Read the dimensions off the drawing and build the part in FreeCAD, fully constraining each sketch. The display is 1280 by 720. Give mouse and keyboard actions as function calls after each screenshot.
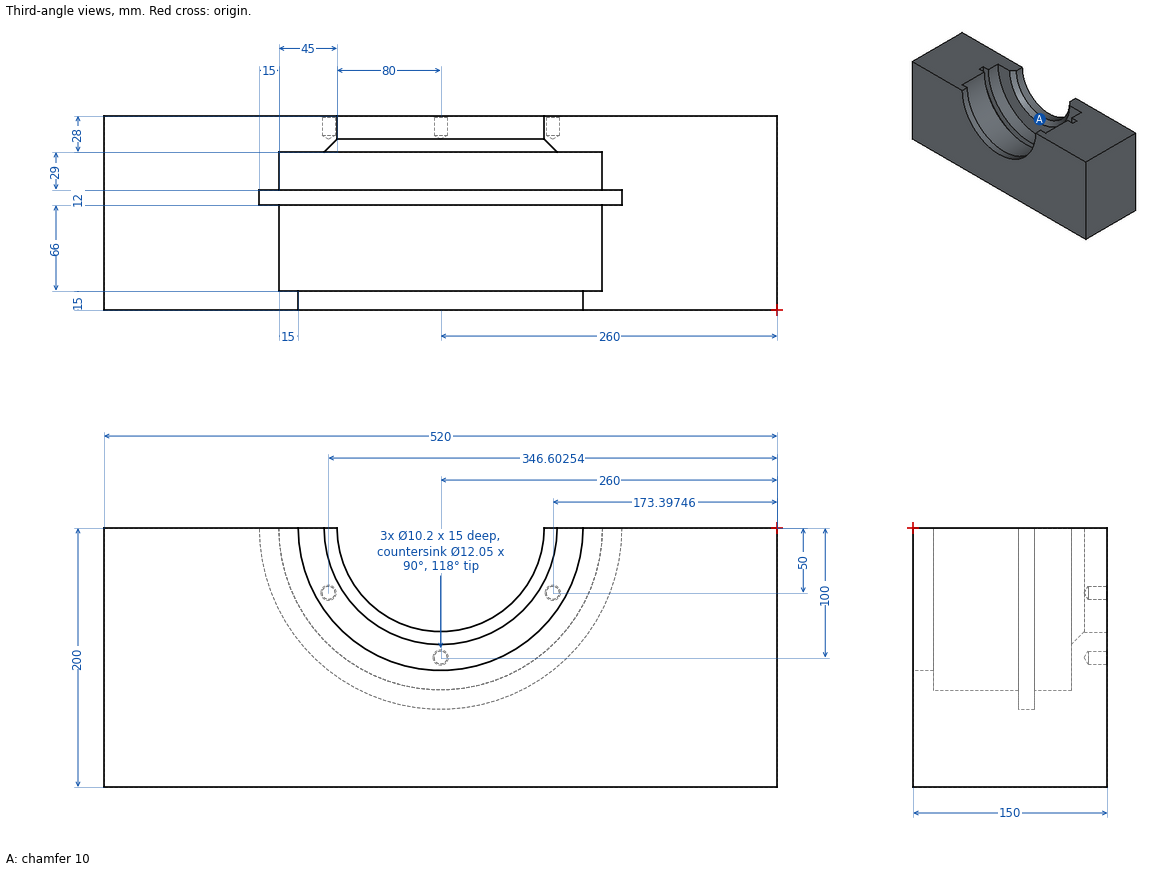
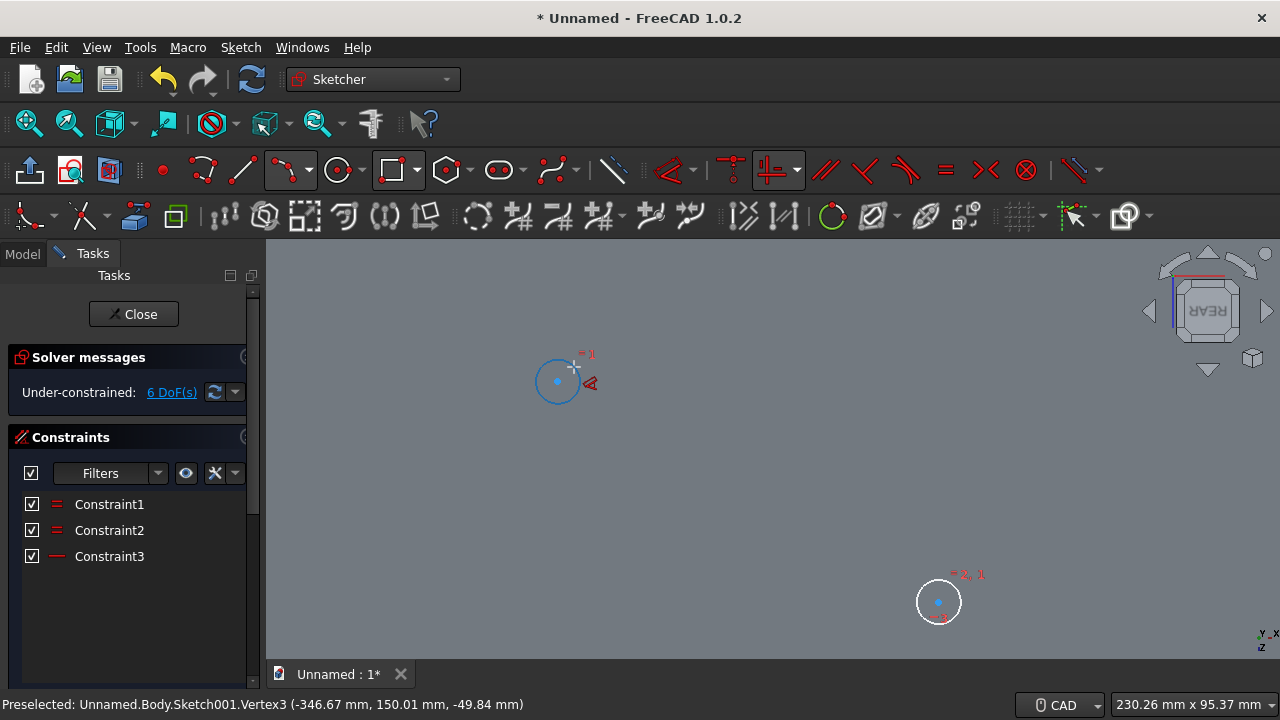
click(574, 366)
click(597, 344)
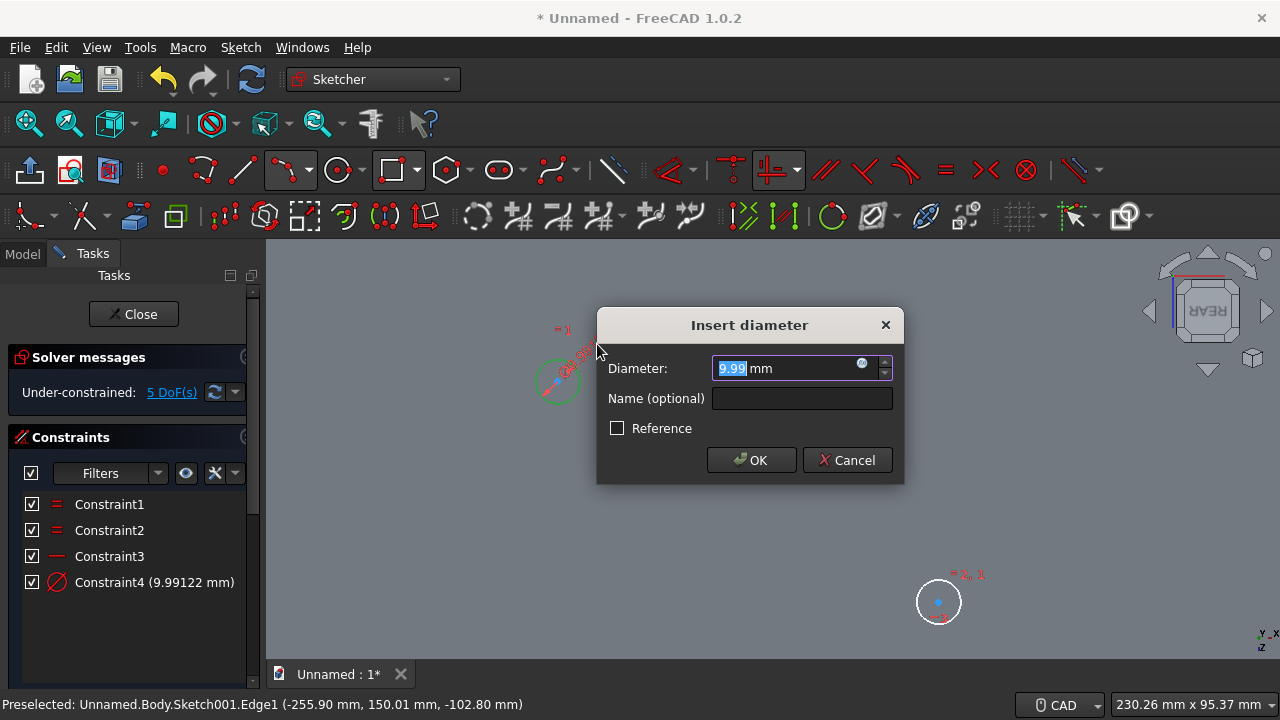
text(10.2)
key(Return)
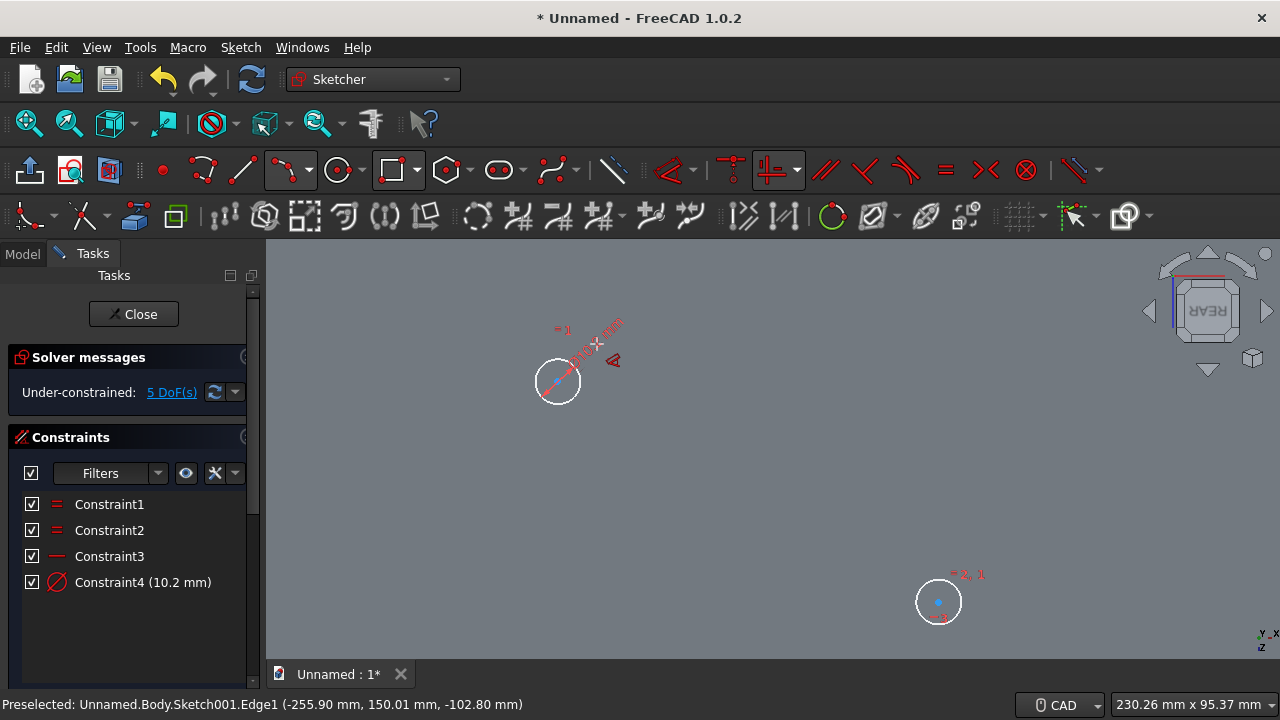
click(939, 602)
click(905, 617)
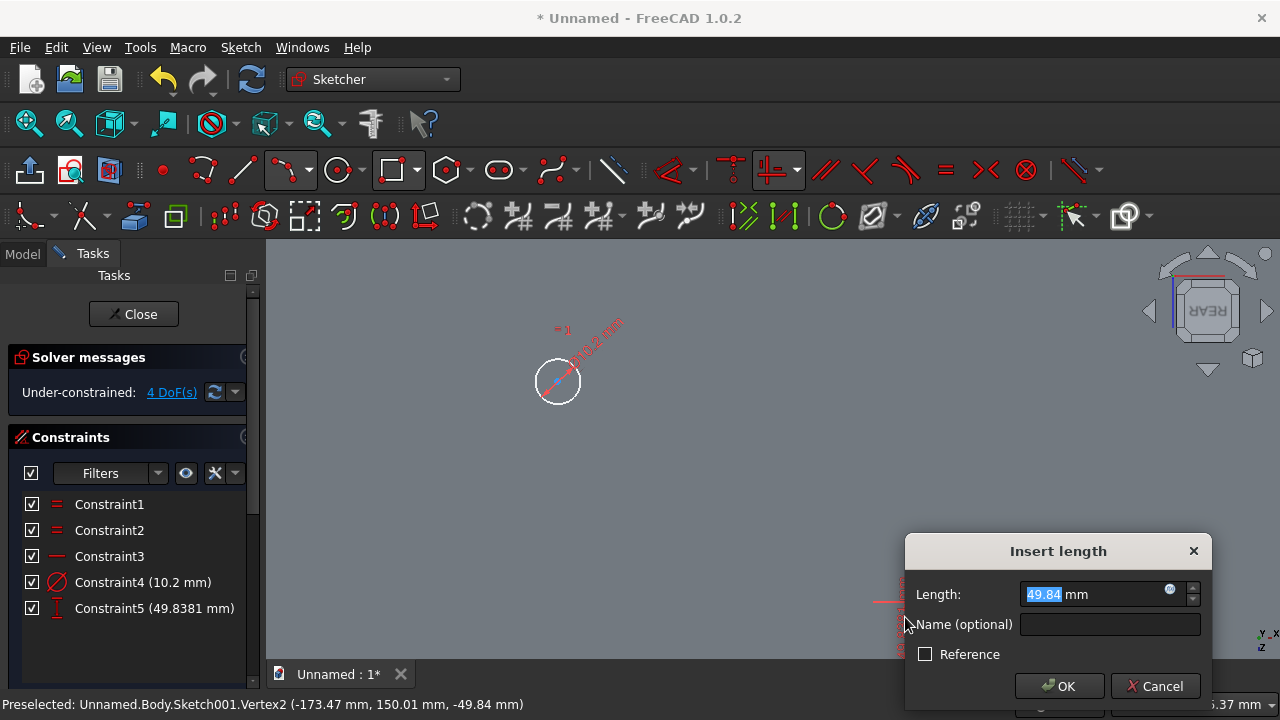
text(50)
key(Return)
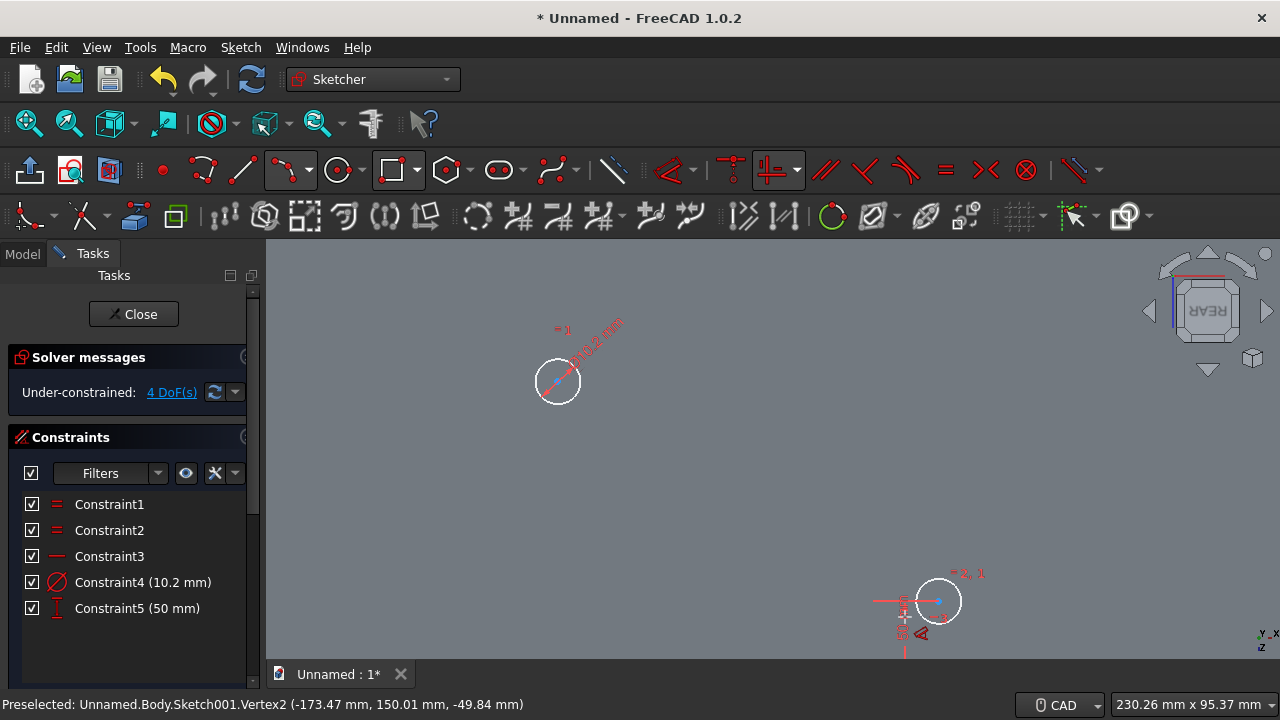
click(558, 382)
click(836, 348)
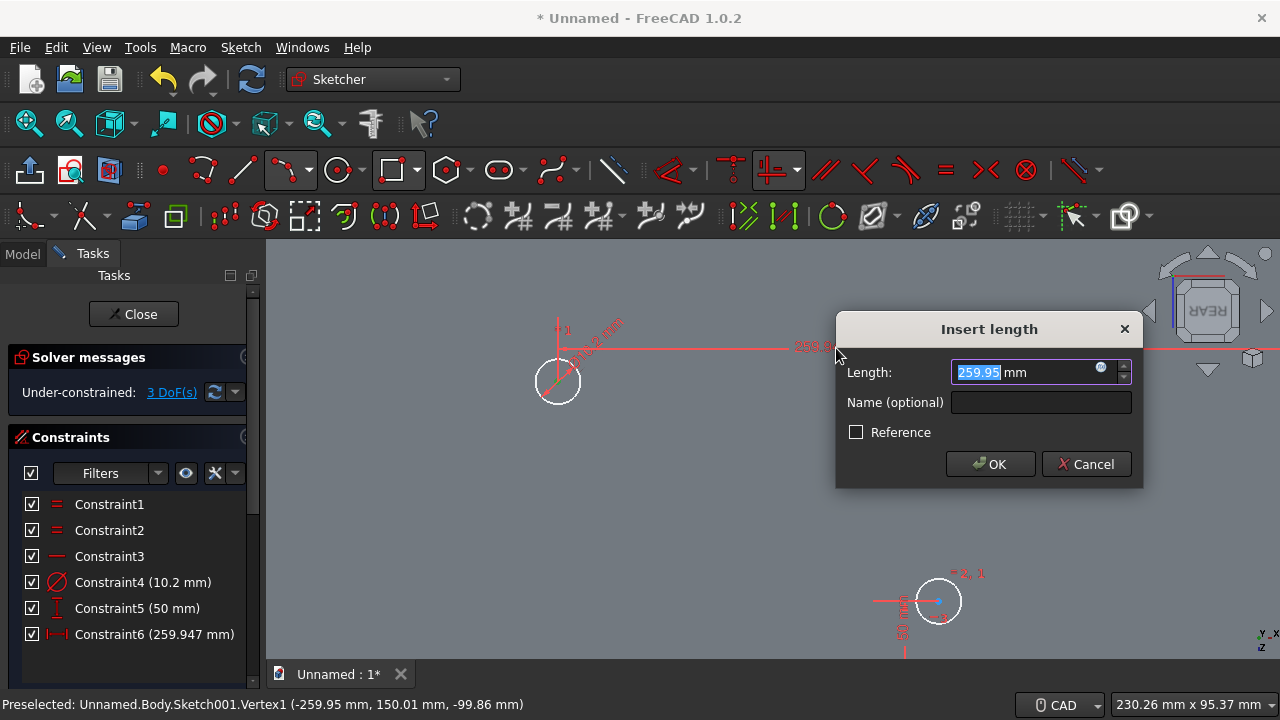
text(260)
key(Return)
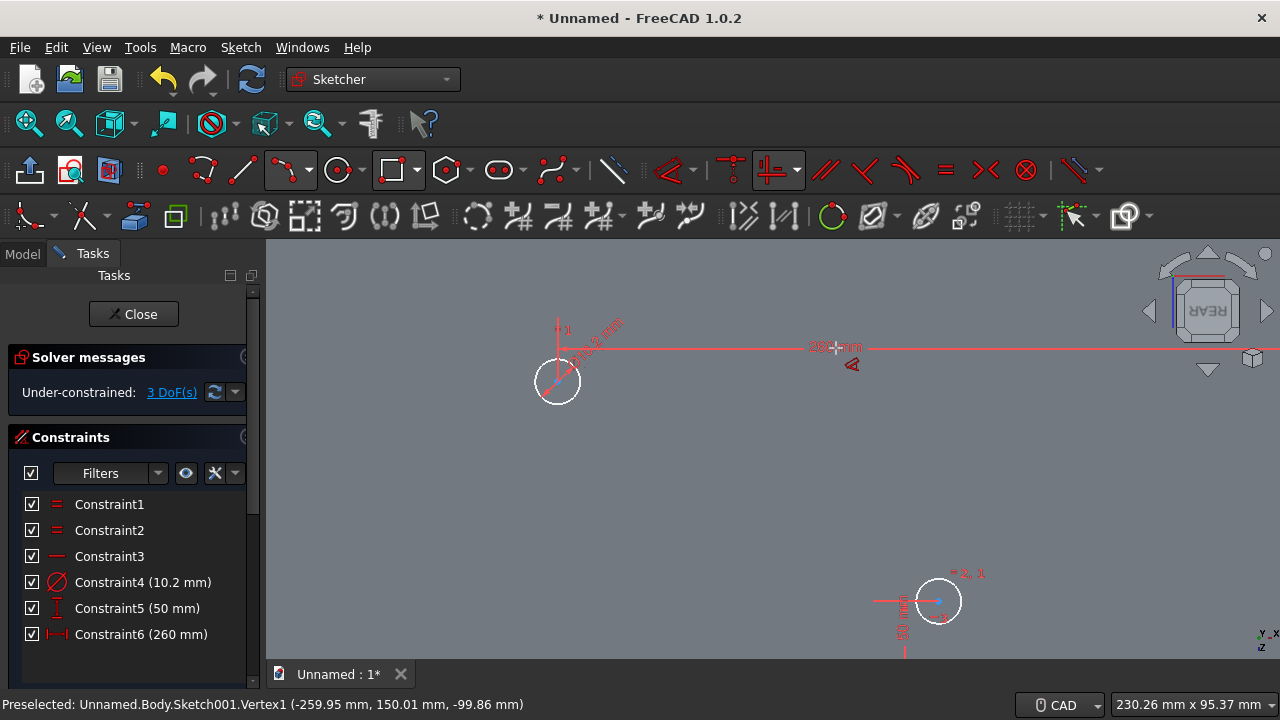
click(558, 382)
click(524, 506)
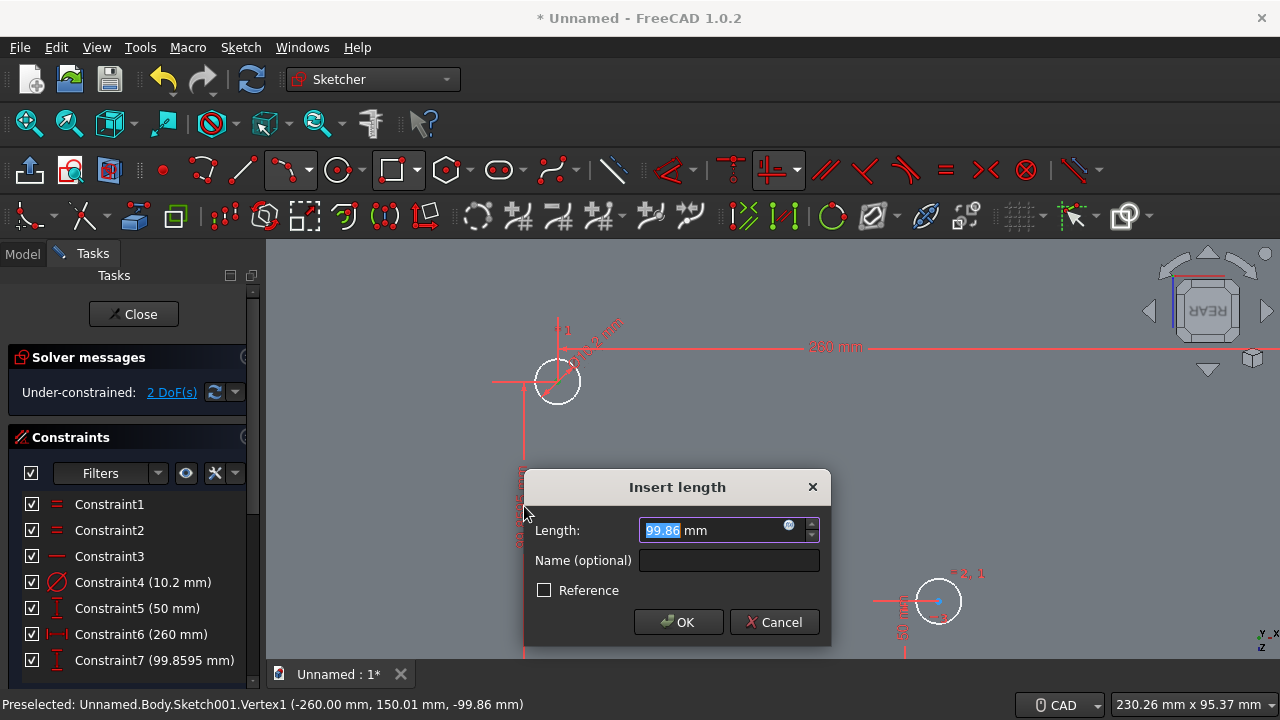
text(100)
key(Return)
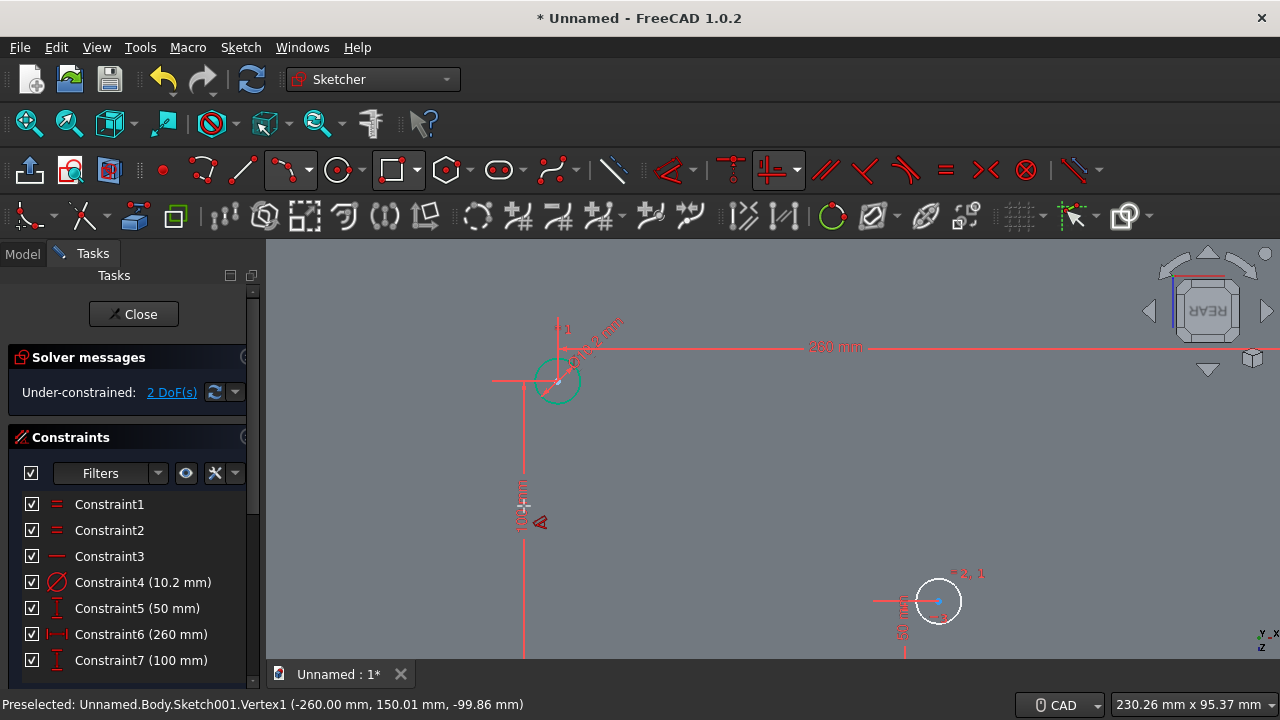
click(939, 601)
click(1027, 567)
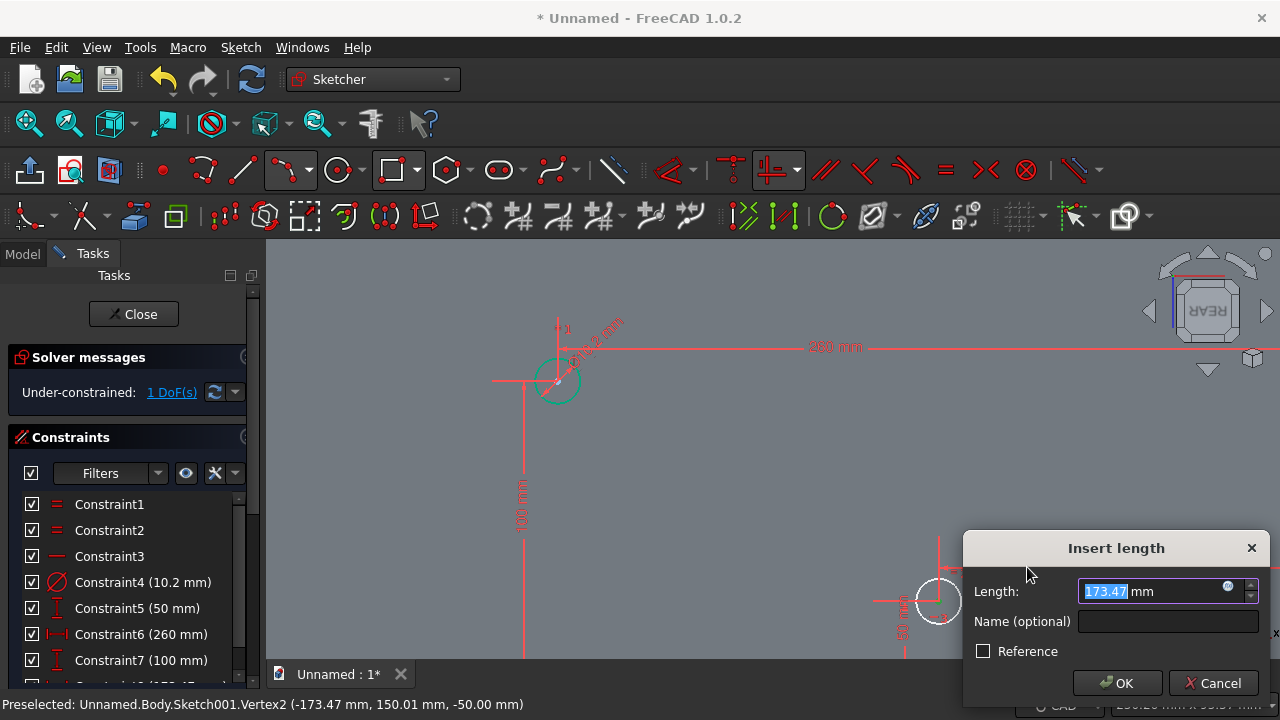
text(173.39746)
key(Return)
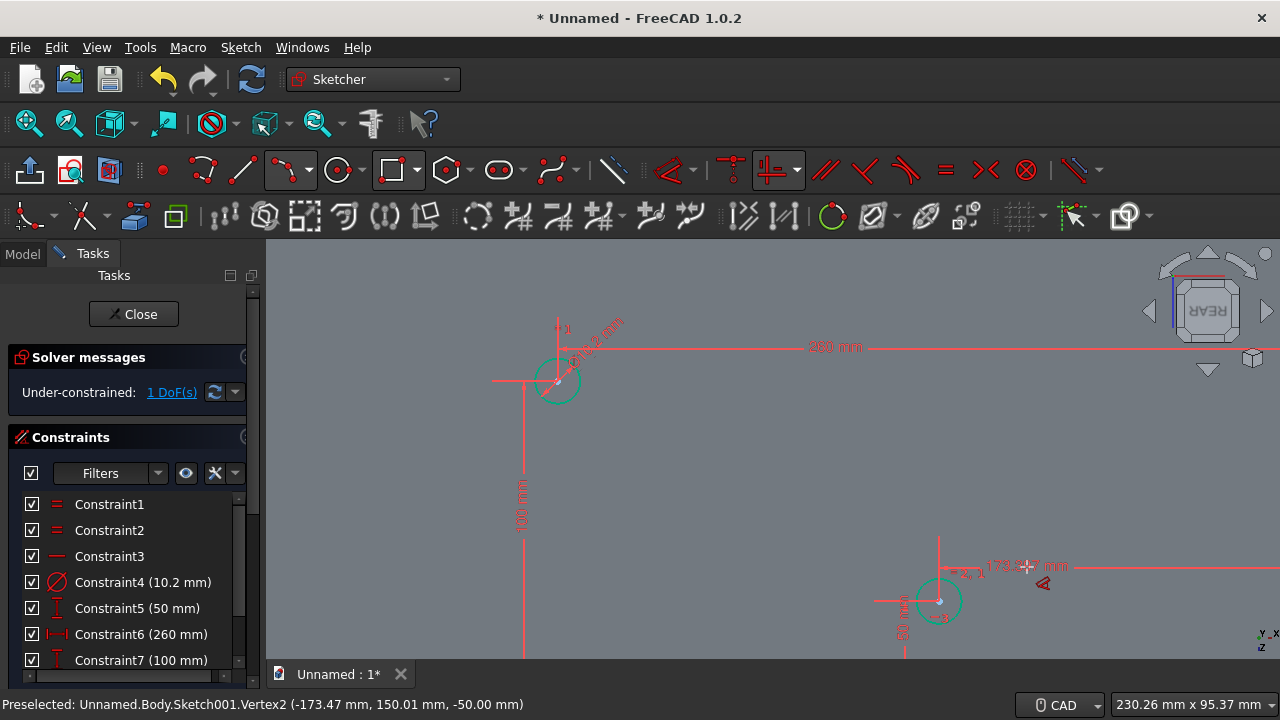
scroll(574, 367, down, 5)